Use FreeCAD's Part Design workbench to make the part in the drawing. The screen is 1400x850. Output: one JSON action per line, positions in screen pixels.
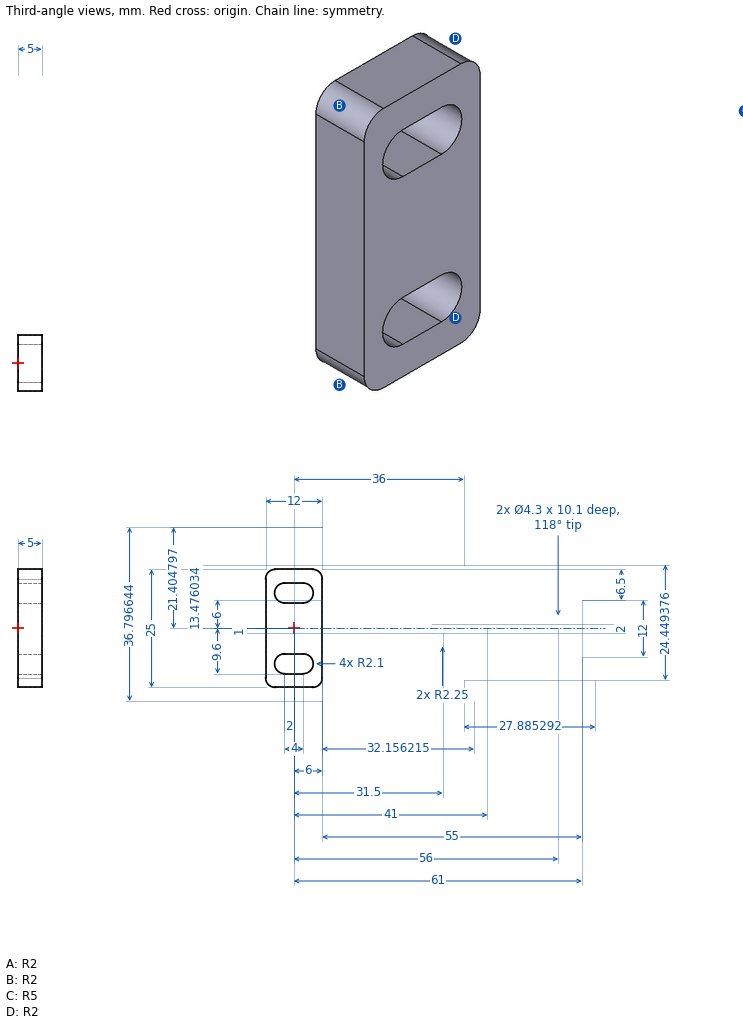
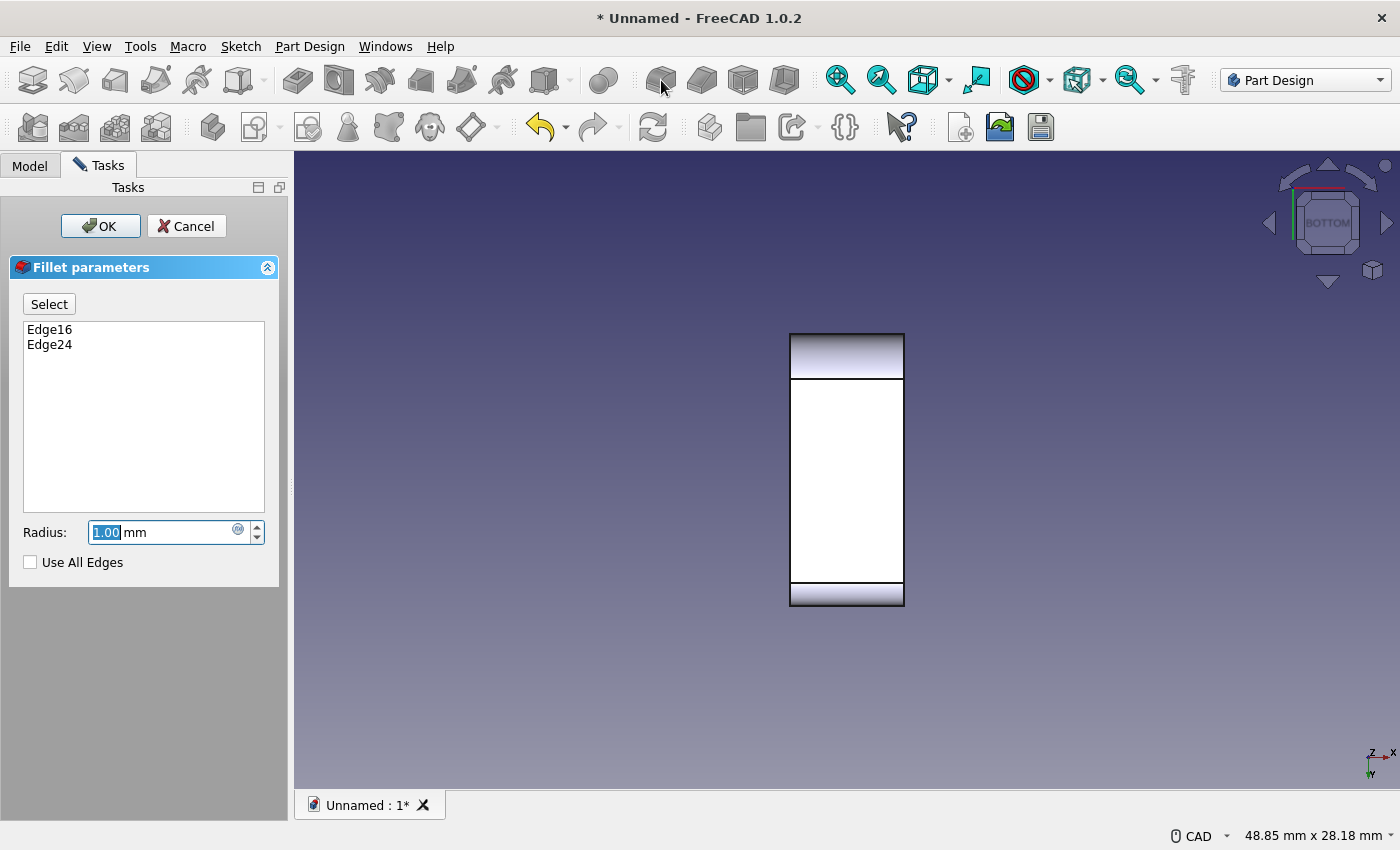
{"action": "type", "text": "2"}
{"action": "key", "text": "Tab"}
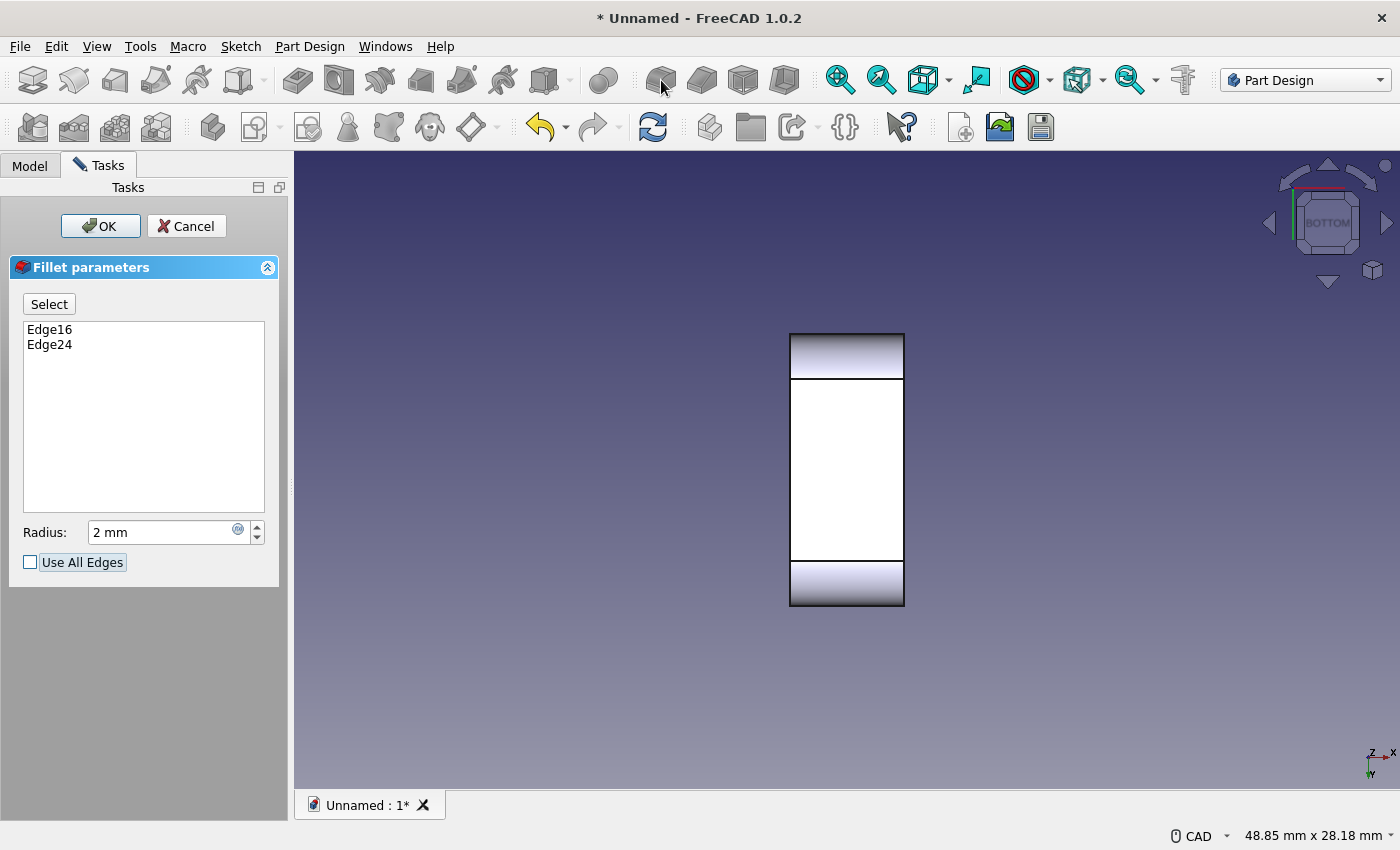
{"action": "left_click", "coordinate": [101, 226]}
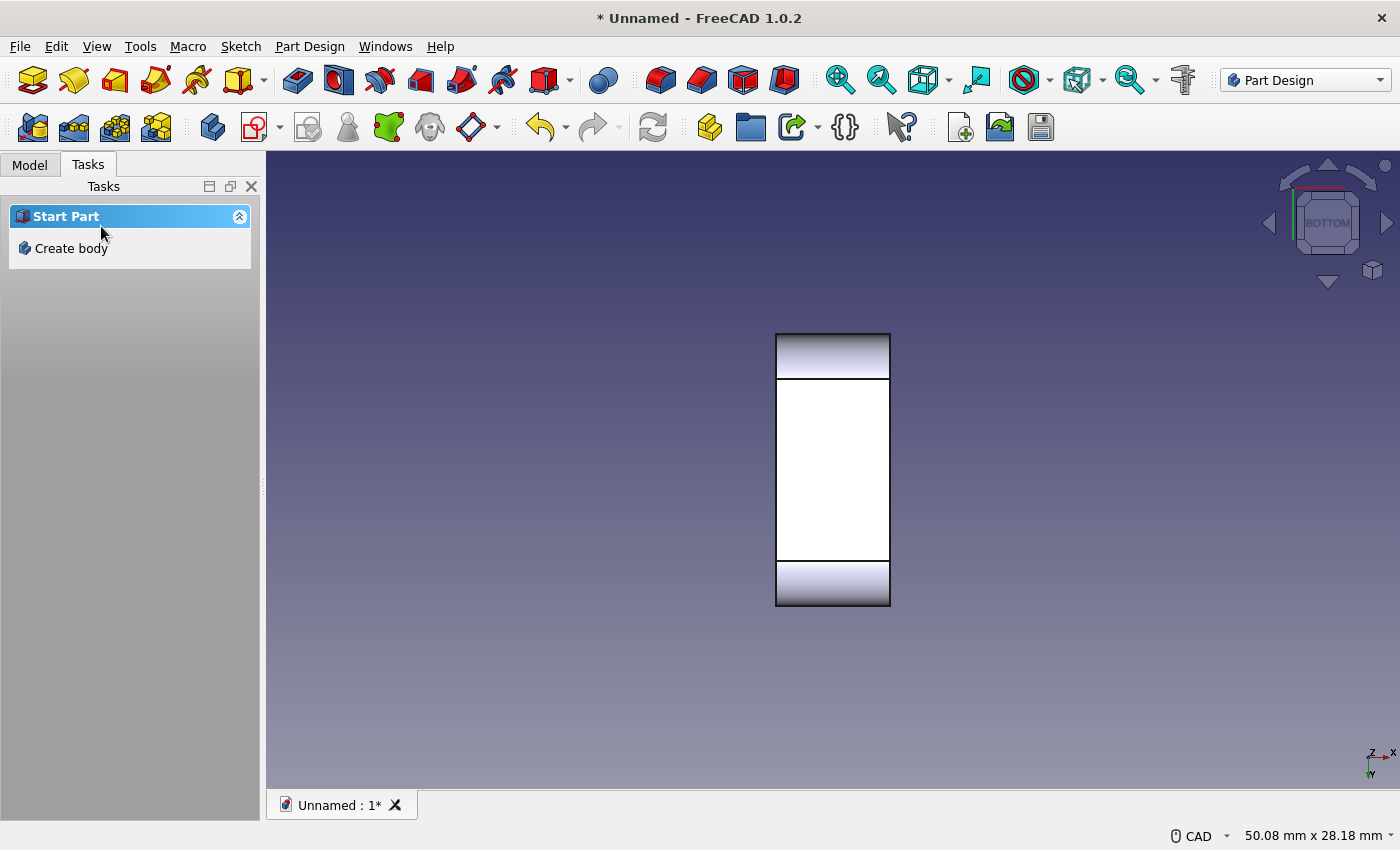
{"action": "key", "text": "0"}